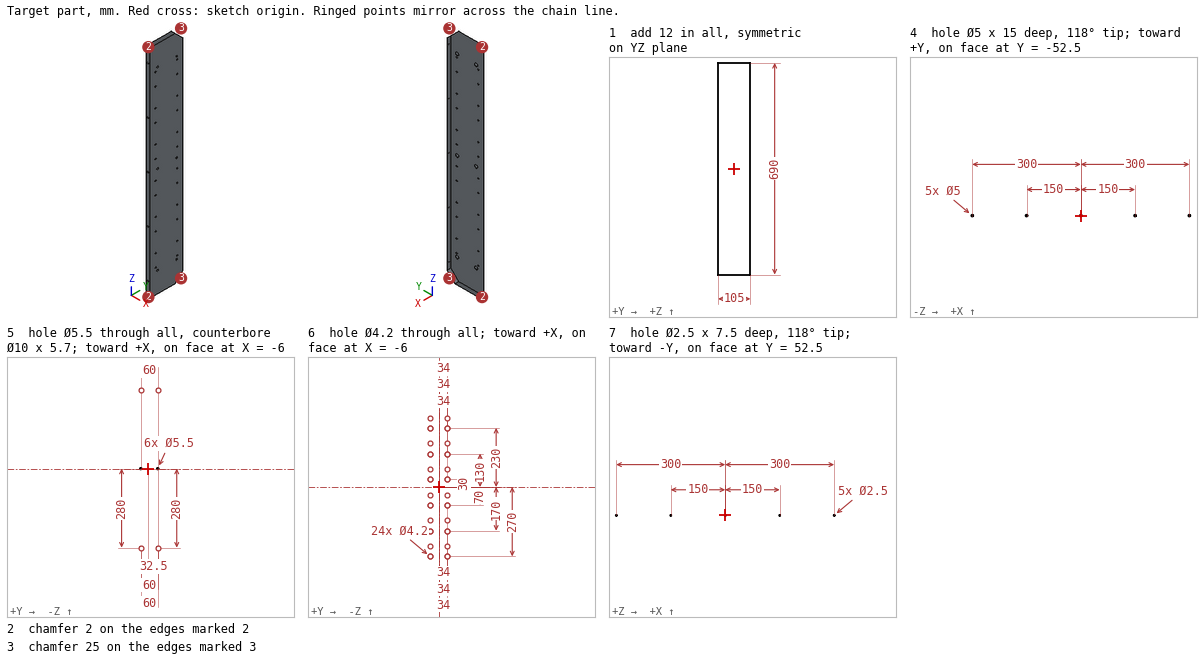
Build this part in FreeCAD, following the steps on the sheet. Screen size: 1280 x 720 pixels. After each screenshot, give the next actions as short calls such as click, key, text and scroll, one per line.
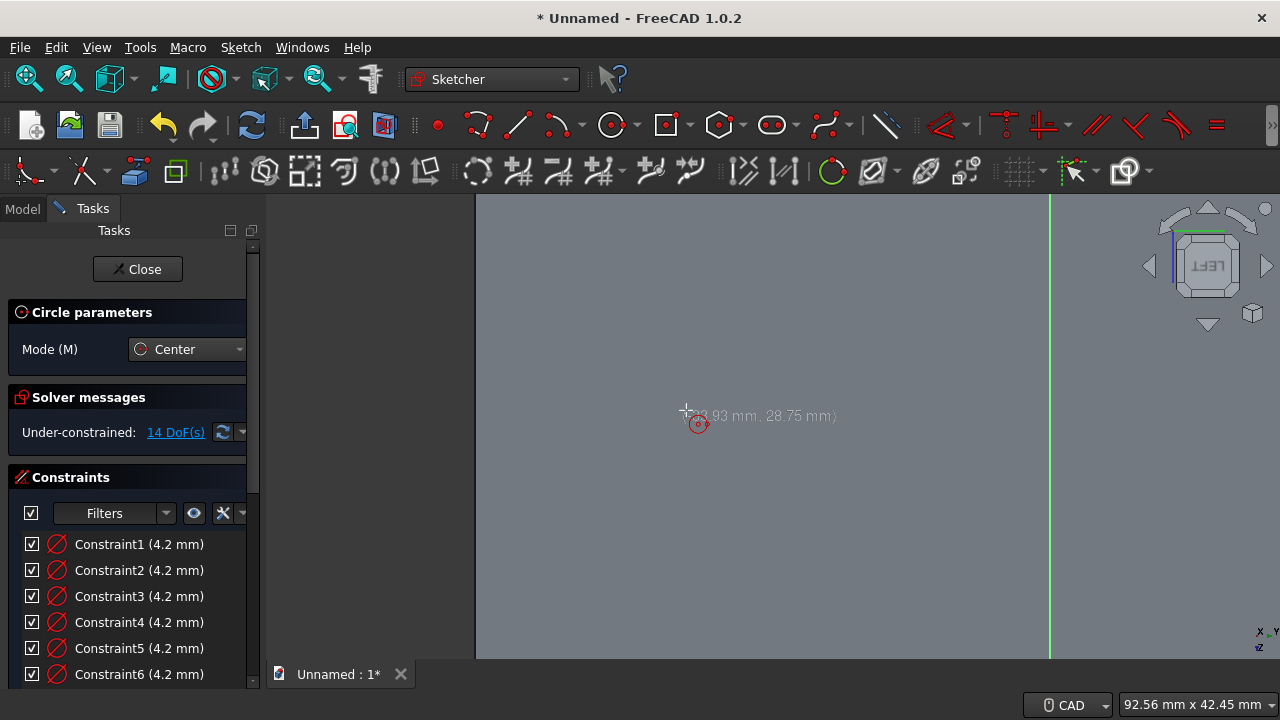
scroll(686, 410, down, 15)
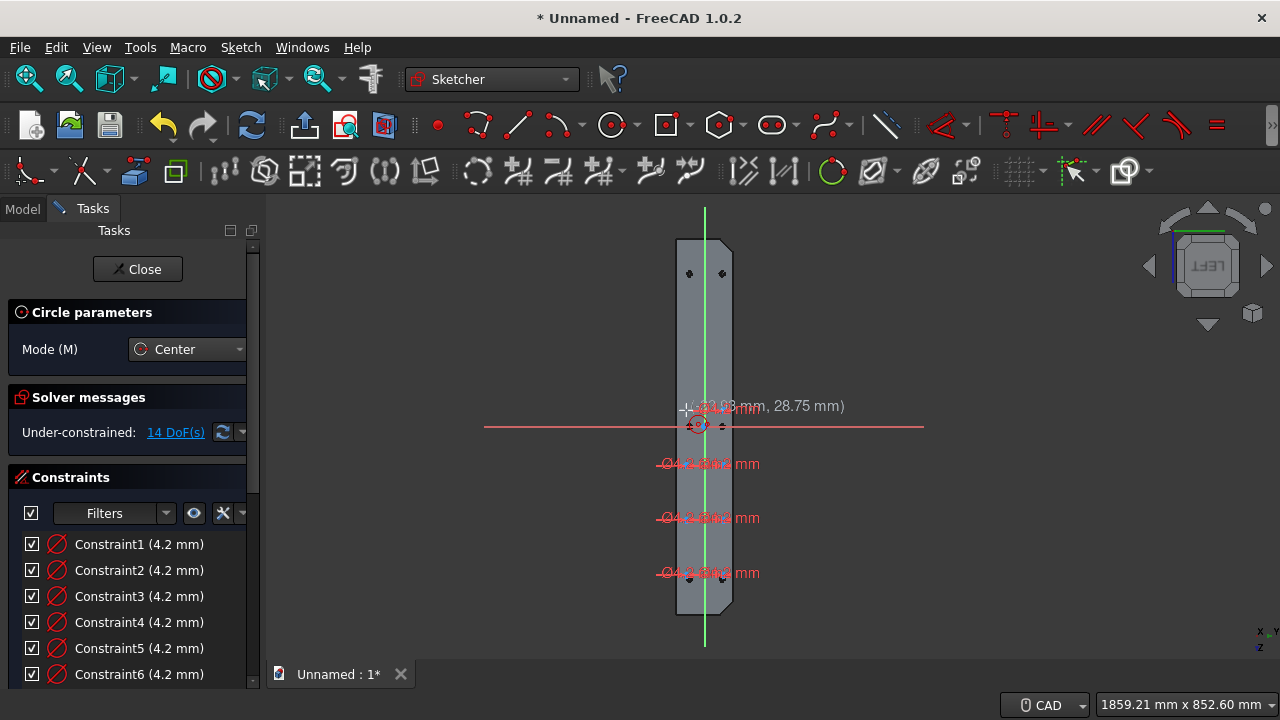
click(686, 410)
move(687, 410)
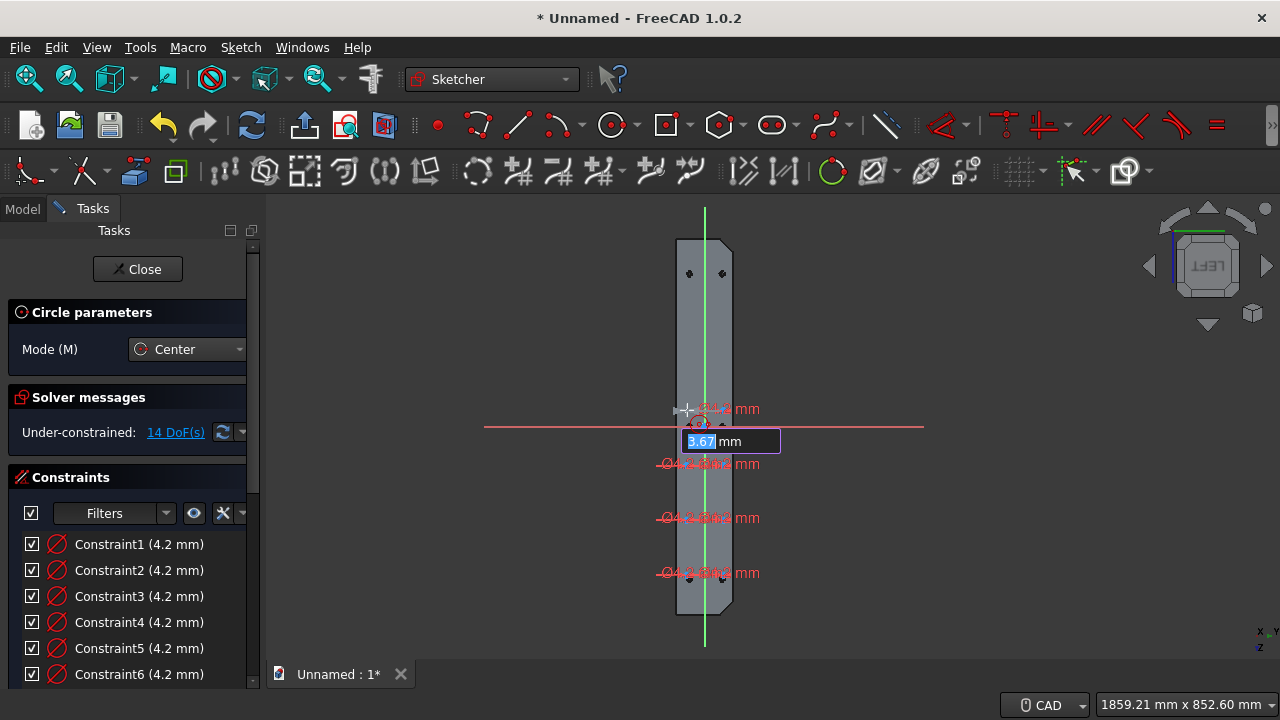
text(4.2)
key(Return)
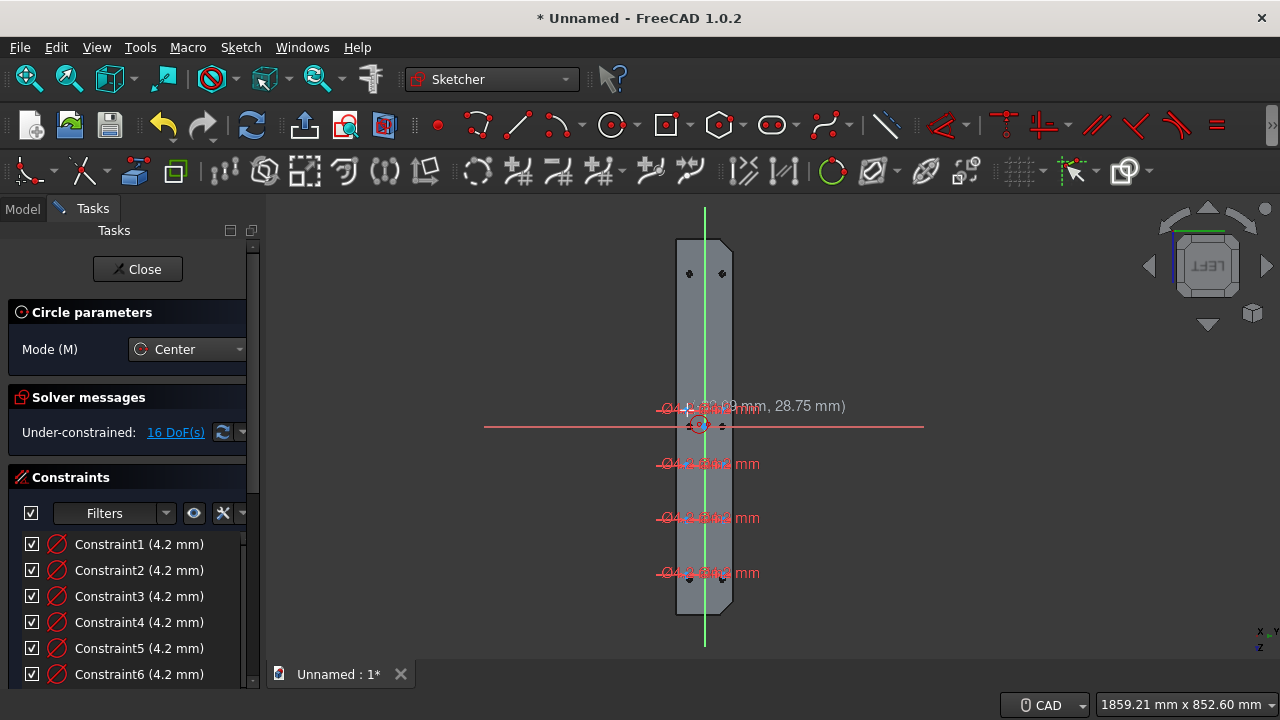
scroll(723, 356, up, 15)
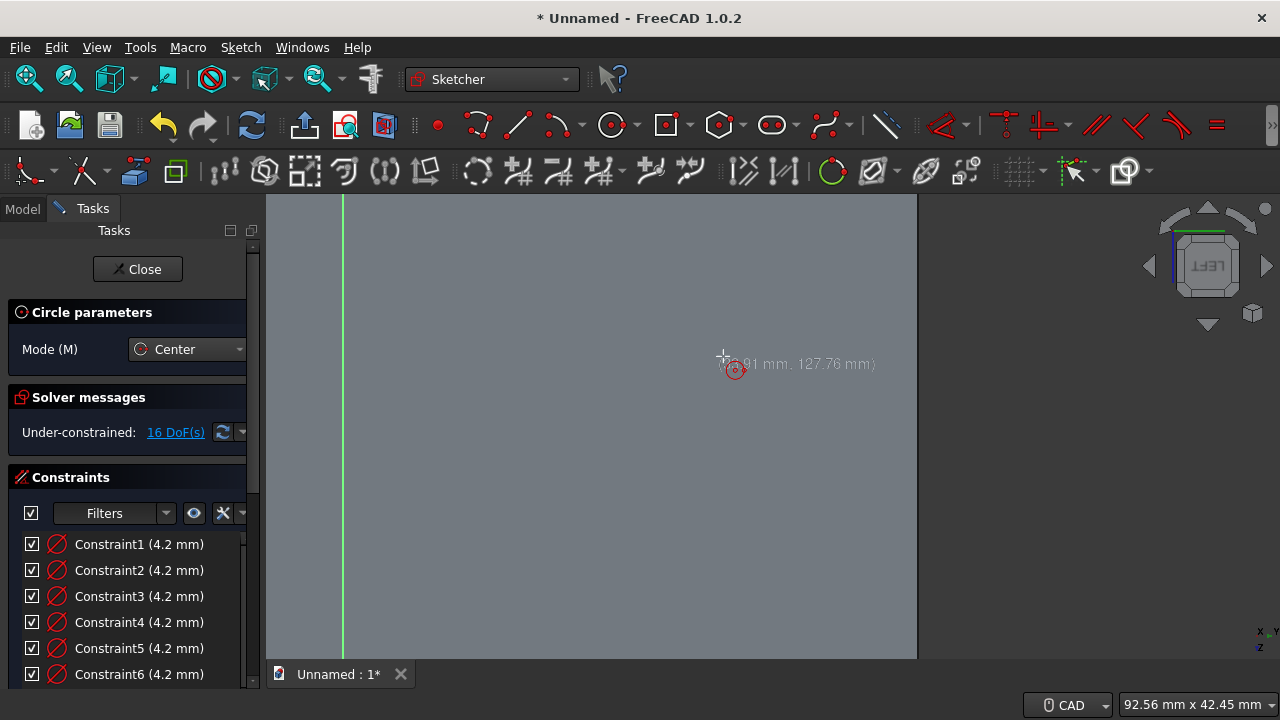
scroll(723, 356, down, 15)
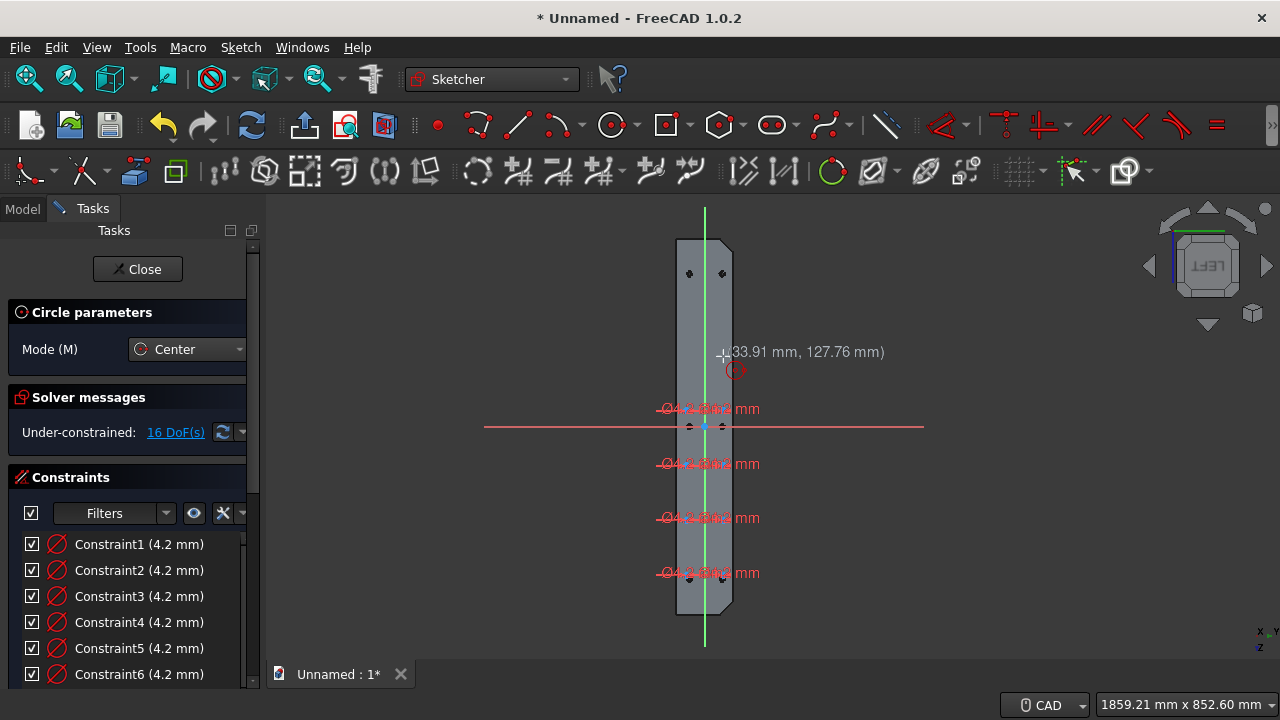
click(723, 356)
move(724, 355)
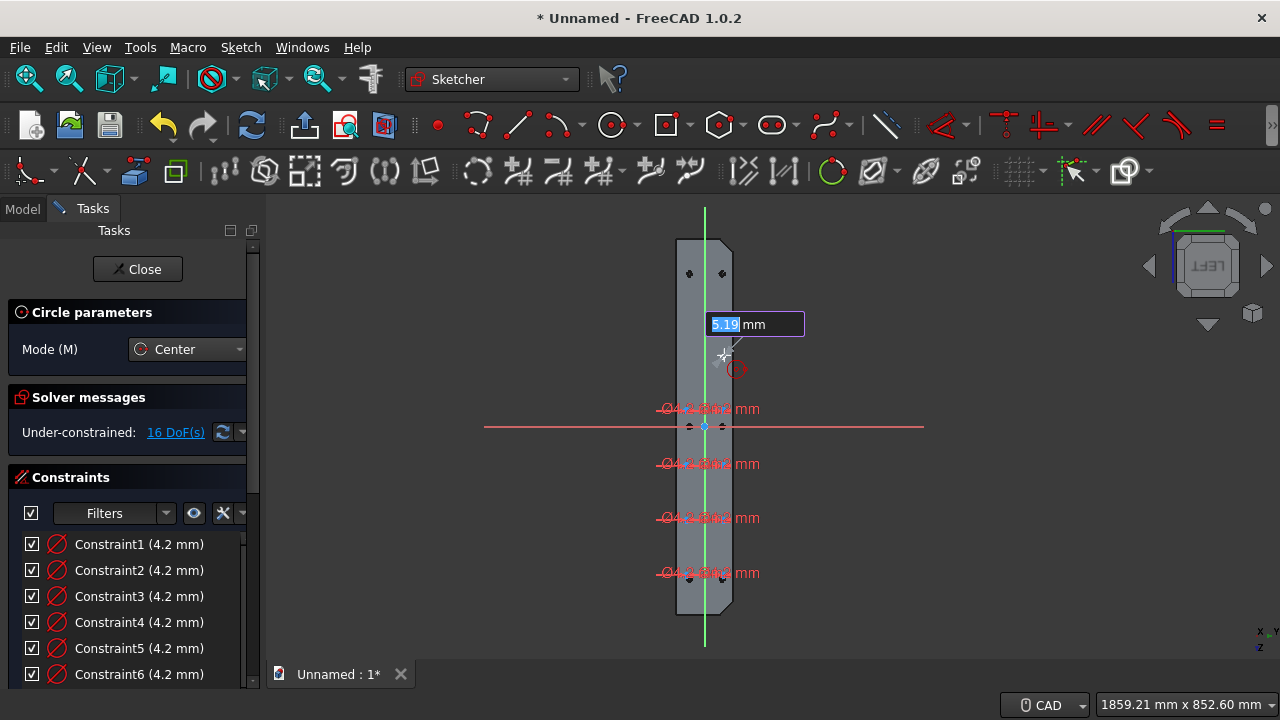
text(4.2)
key(Return)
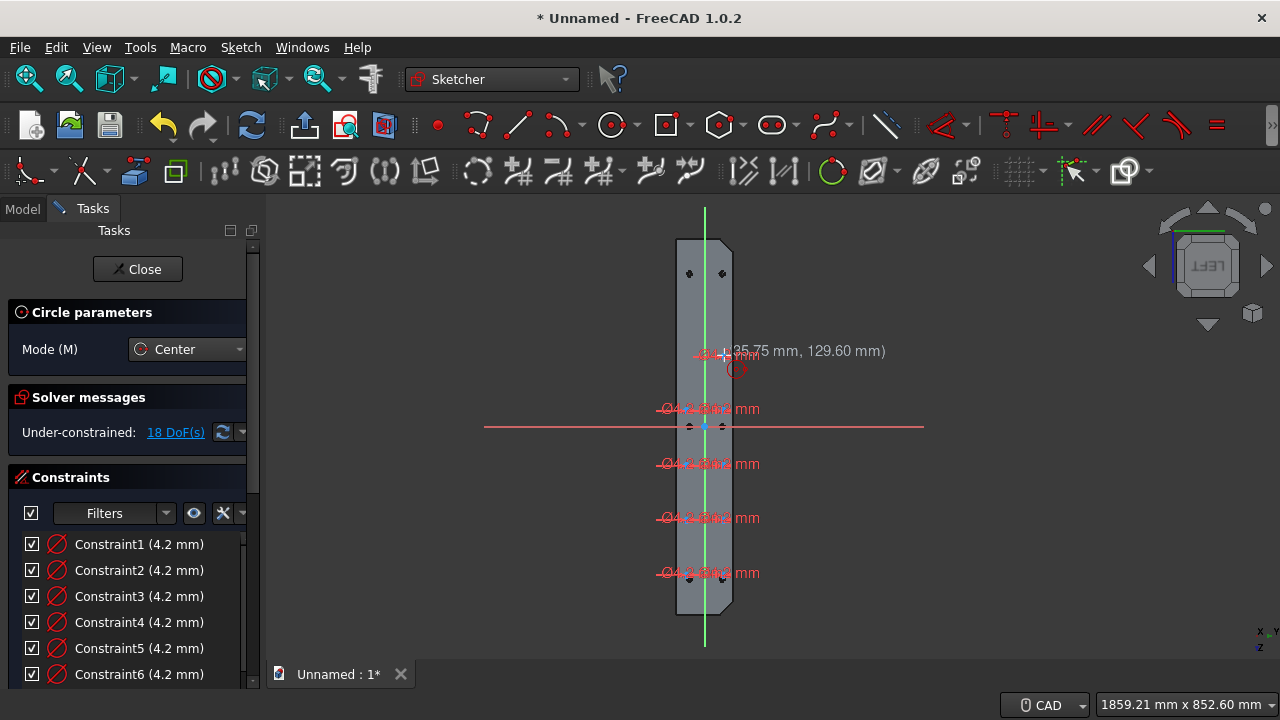
scroll(686, 356, up, 15)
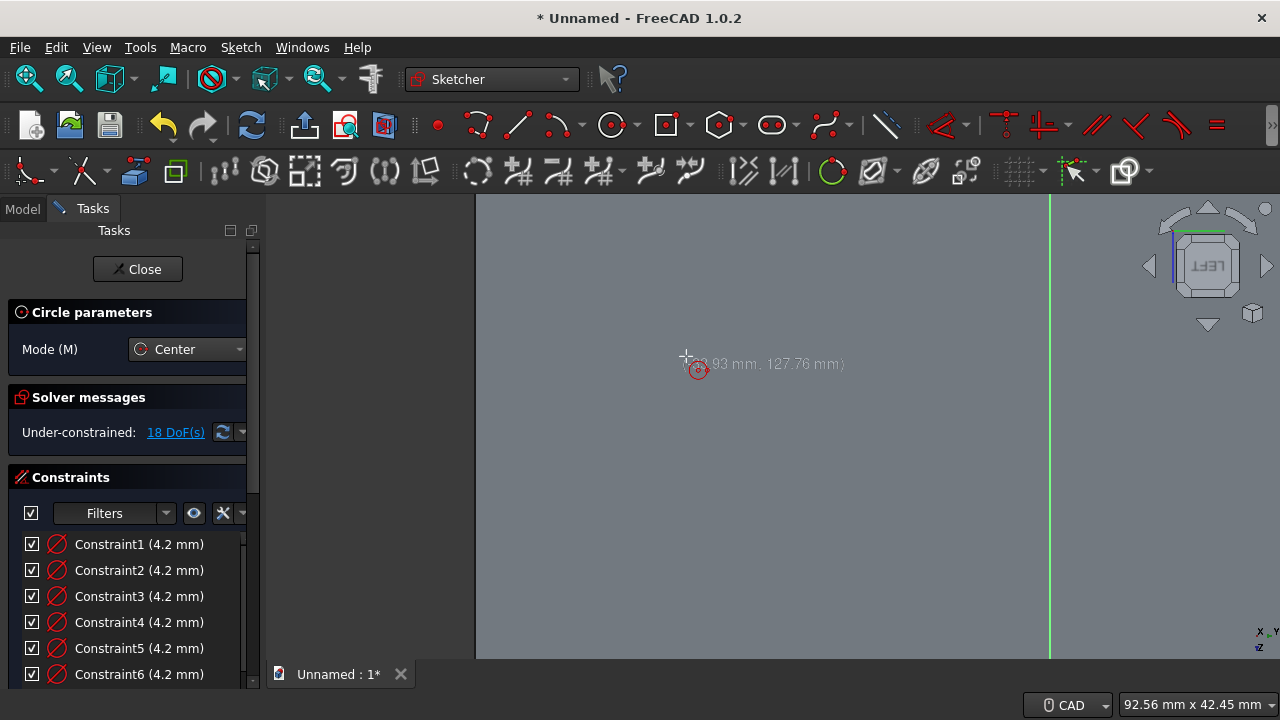
scroll(686, 356, down, 15)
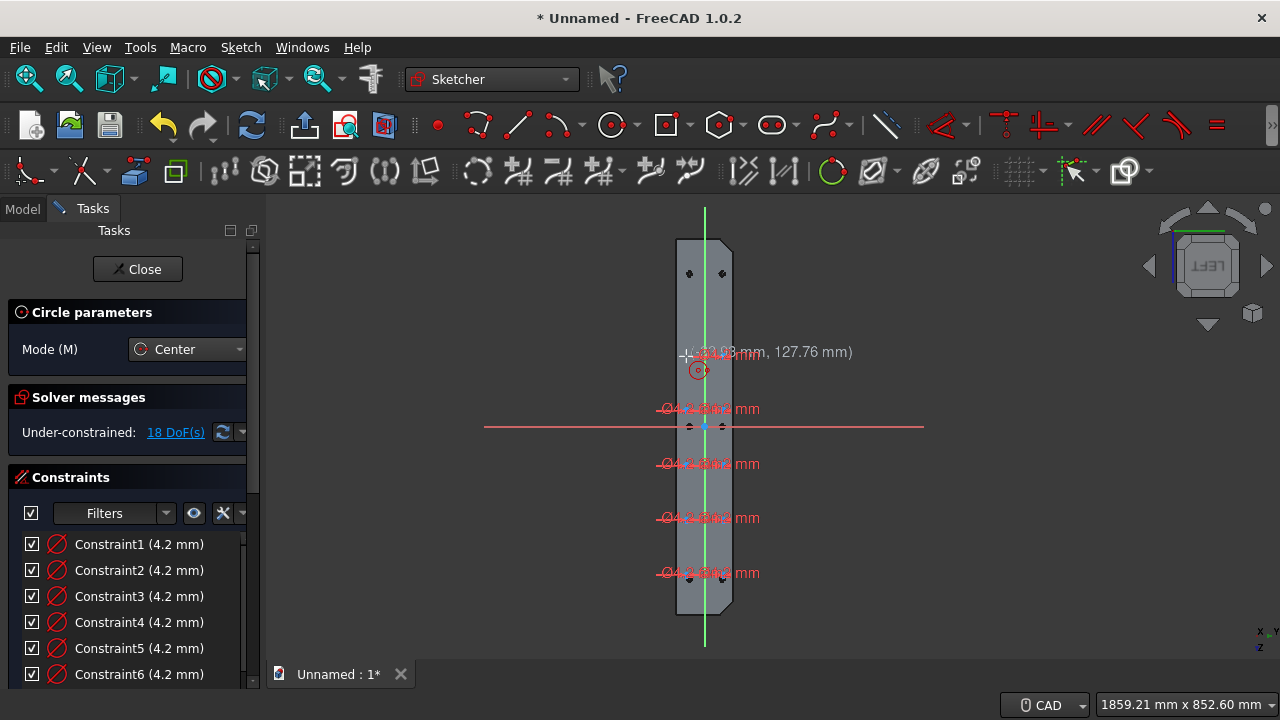
click(686, 356)
move(687, 355)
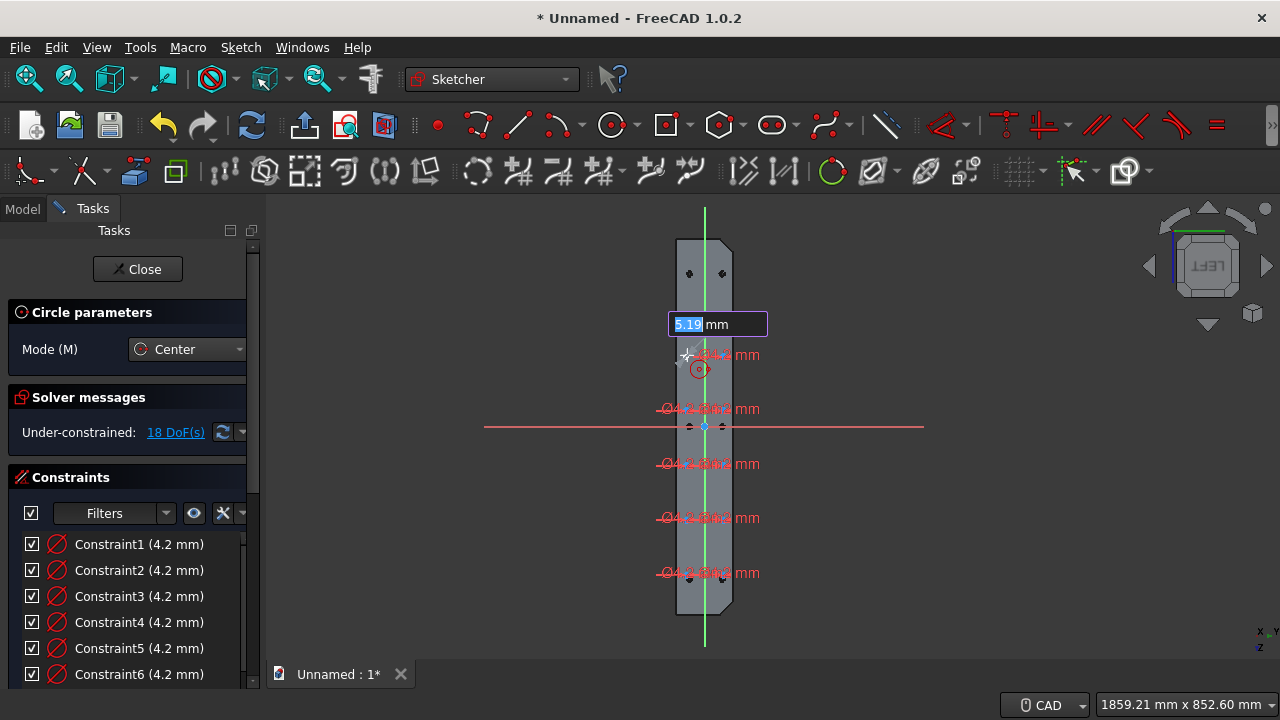
text(4.2)
key(Return)